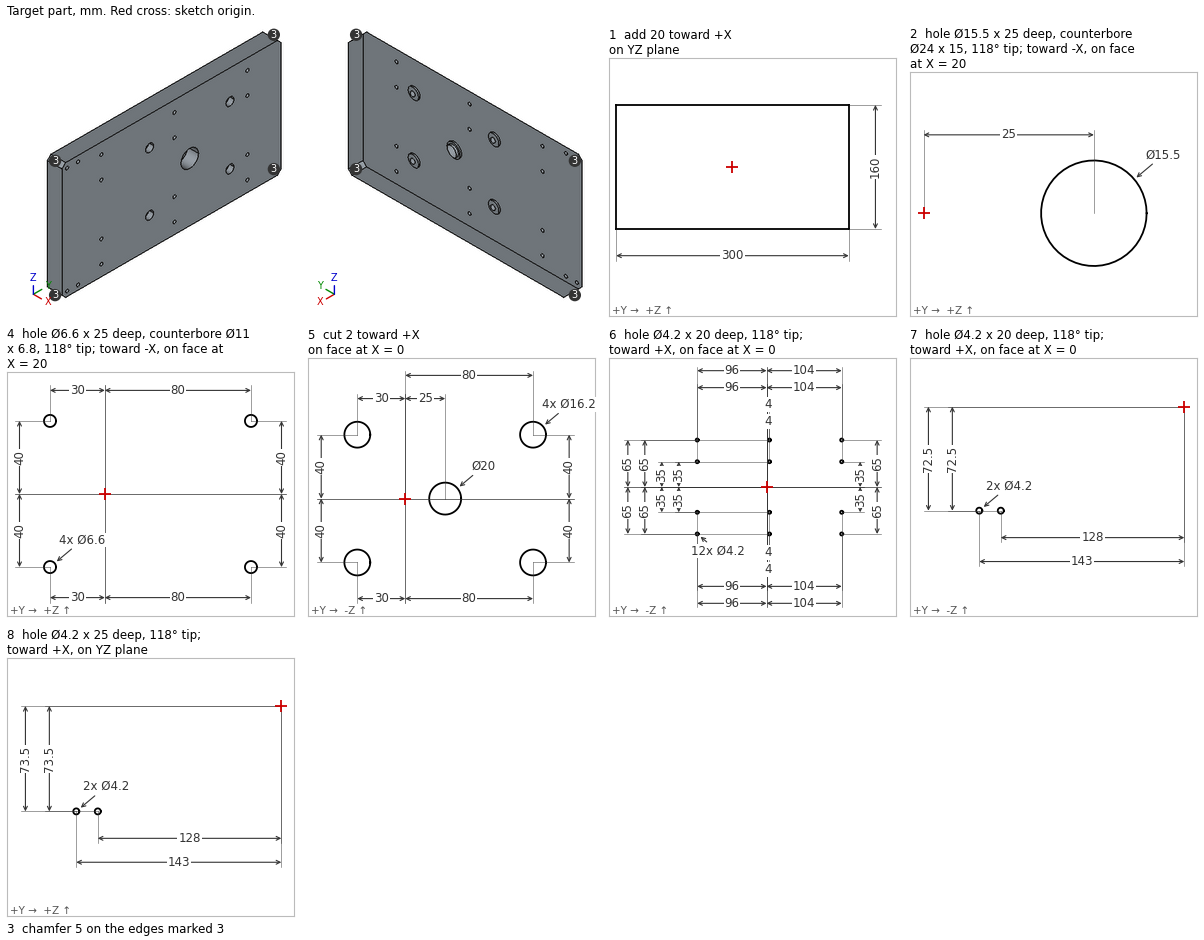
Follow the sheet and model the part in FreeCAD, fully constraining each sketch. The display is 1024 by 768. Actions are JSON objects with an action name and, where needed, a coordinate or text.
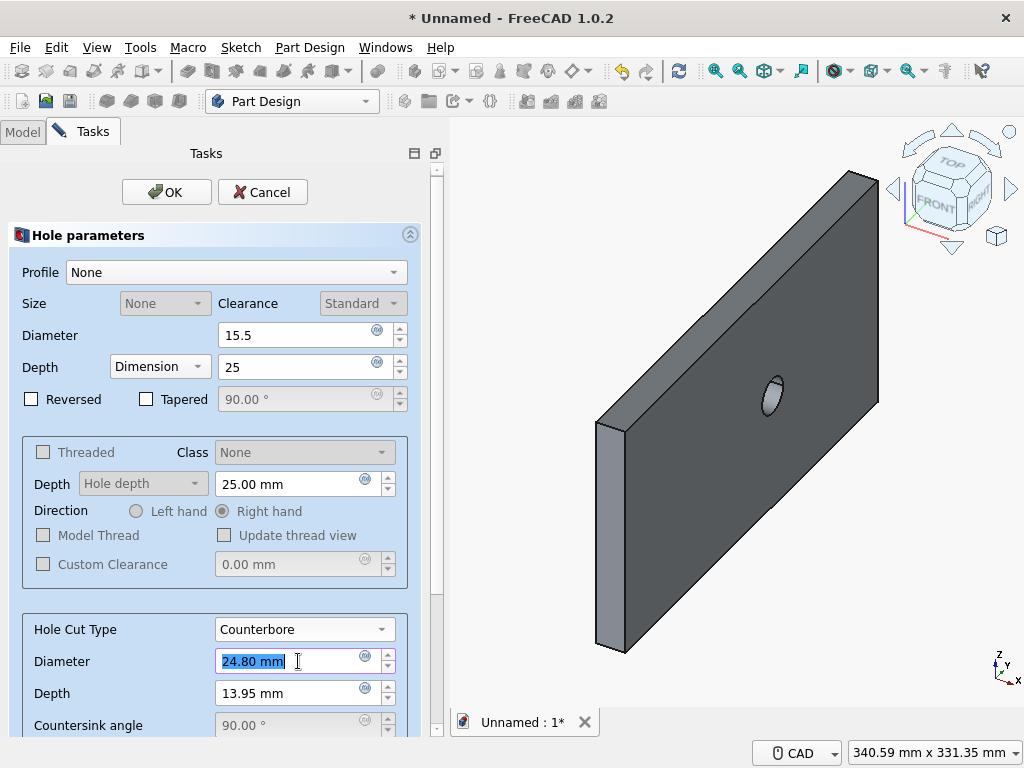
{"action": "type", "text": "24"}
{"action": "key", "text": "Tab"}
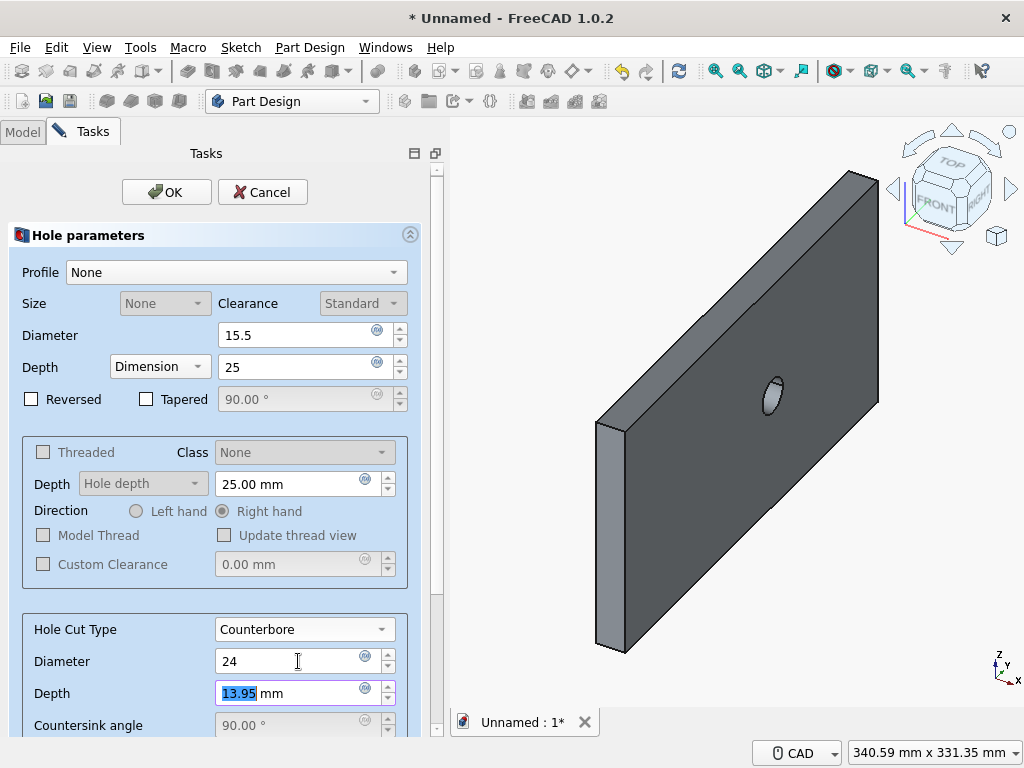
{"action": "type", "text": "15"}
{"action": "key", "text": "Tab"}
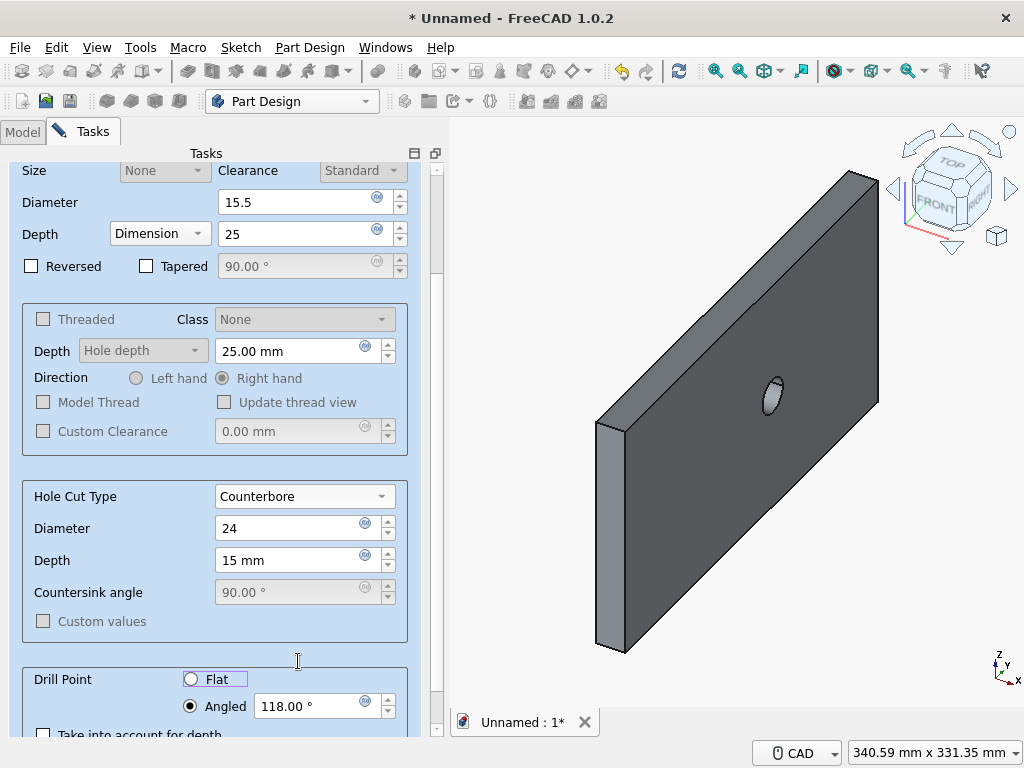
{"action": "scroll", "coordinate": [437, 450], "scroll_direction": "up", "scroll_amount": 3}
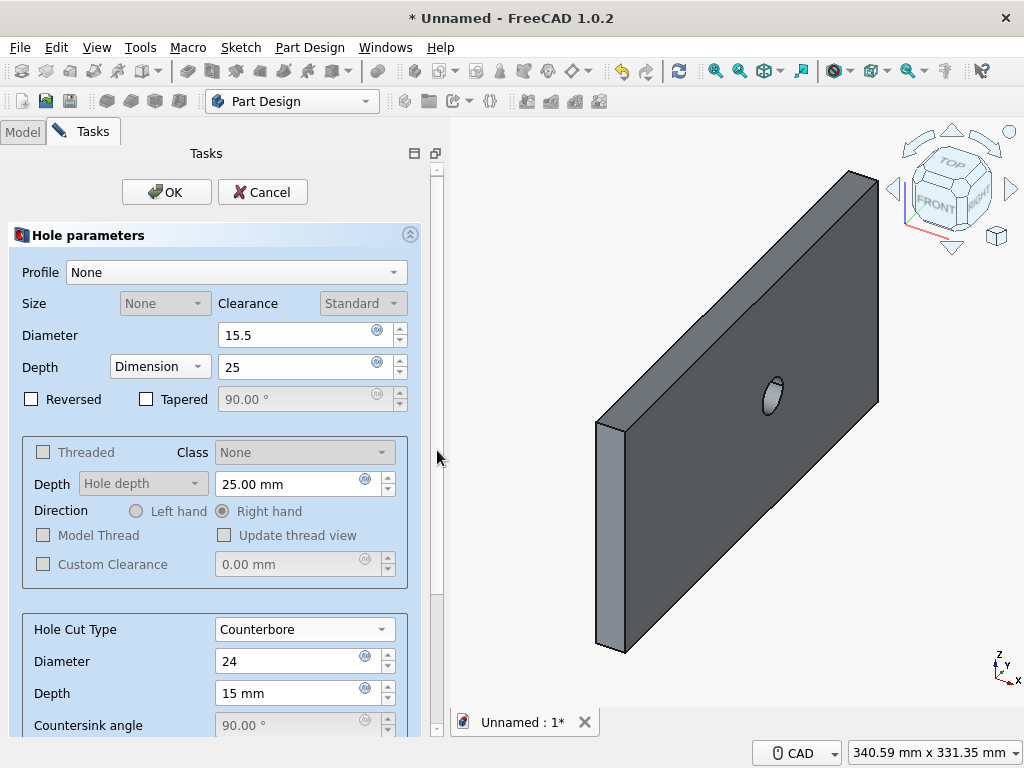
{"action": "left_click", "coordinate": [167, 192]}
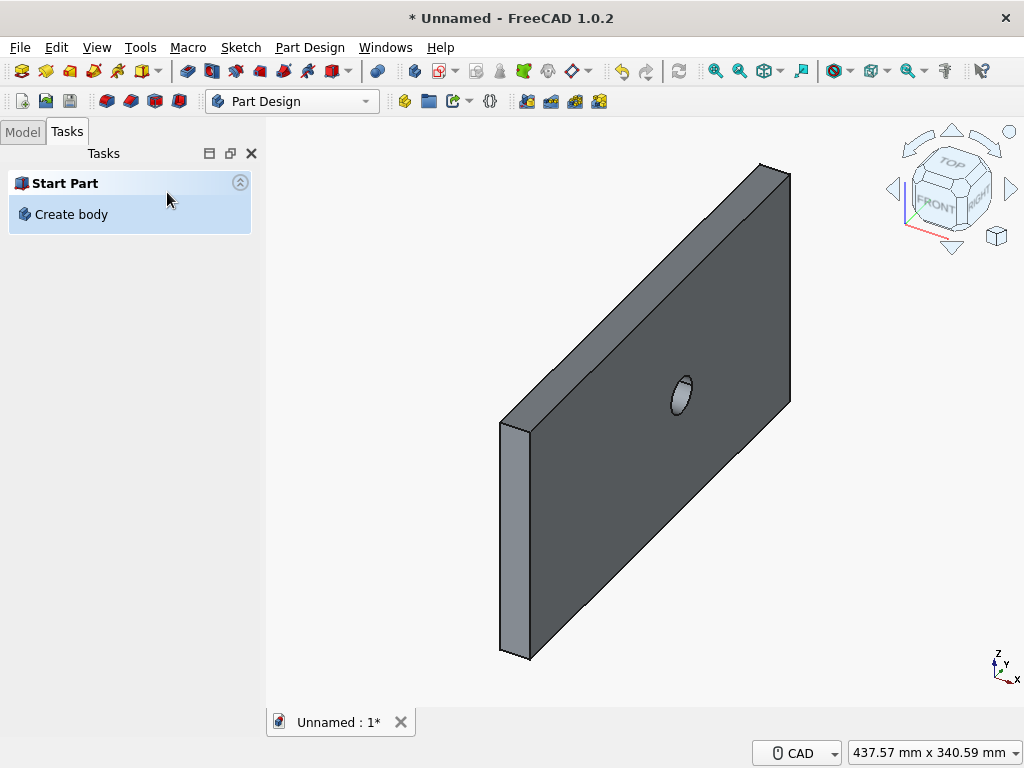
{"action": "left_click", "coordinate": [515, 427]}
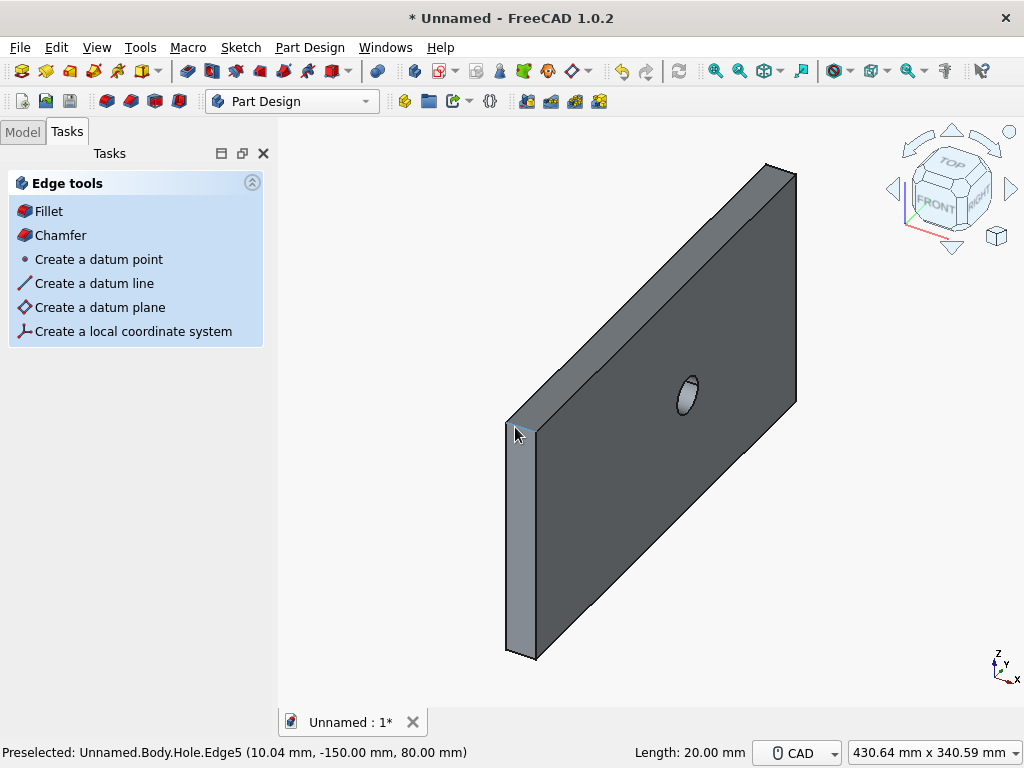
{"action": "key", "text": "0"}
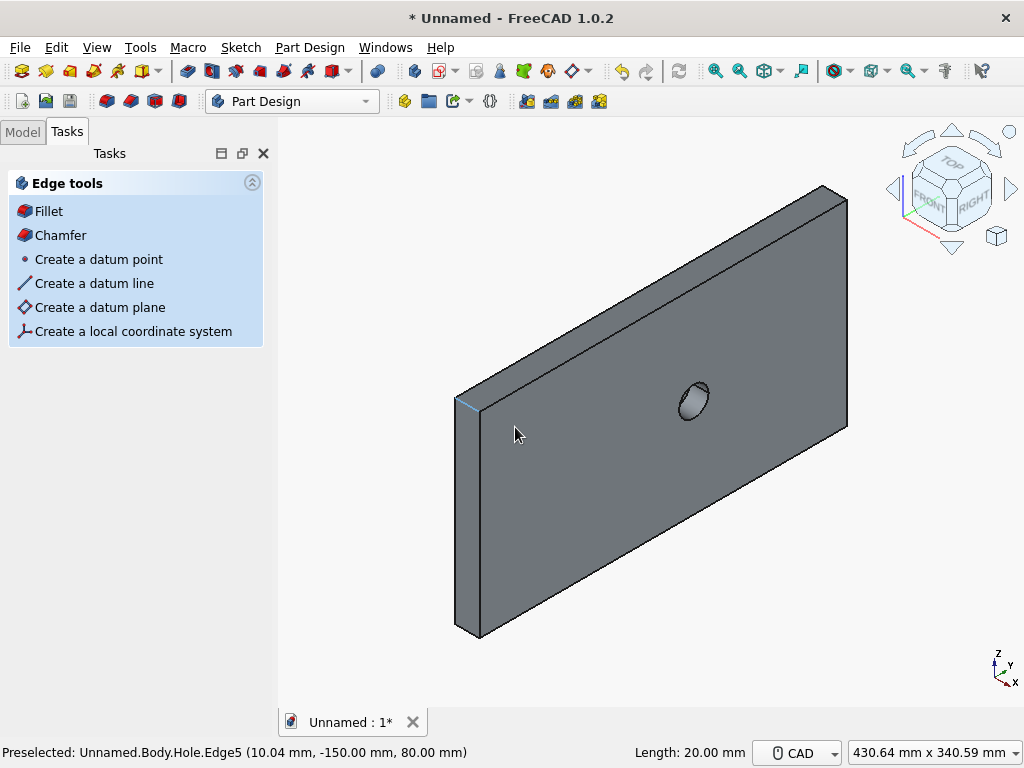
{"action": "key", "text": "2"}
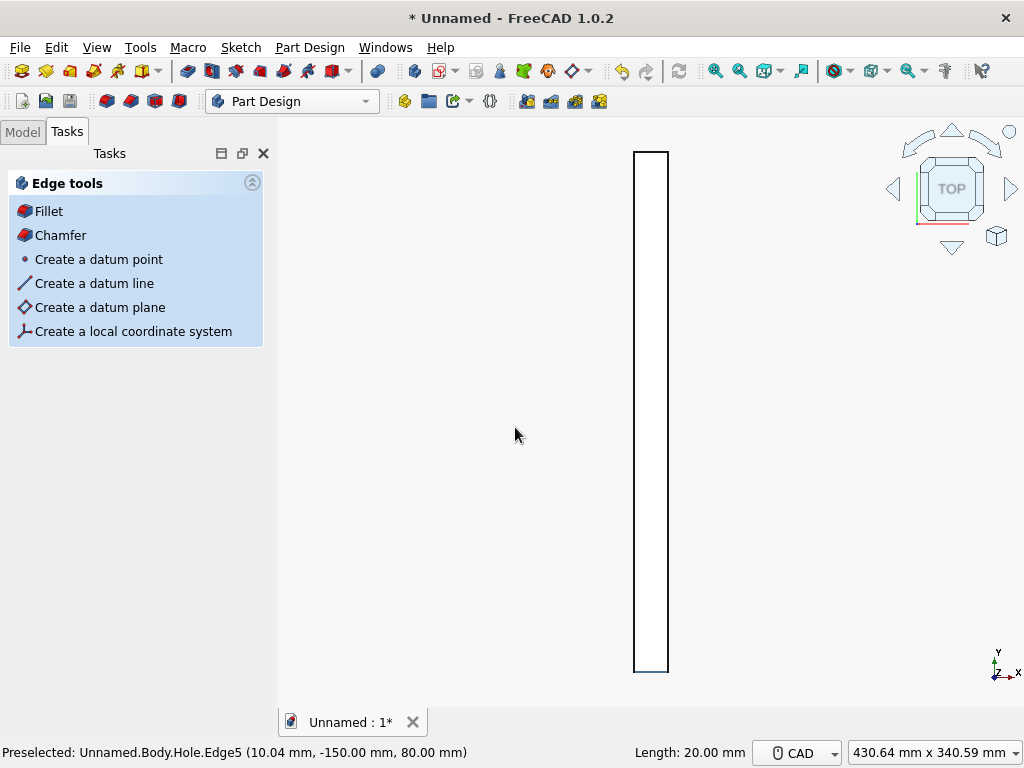
{"action": "left_click", "coordinate": [651, 151], "text": "ctrl"}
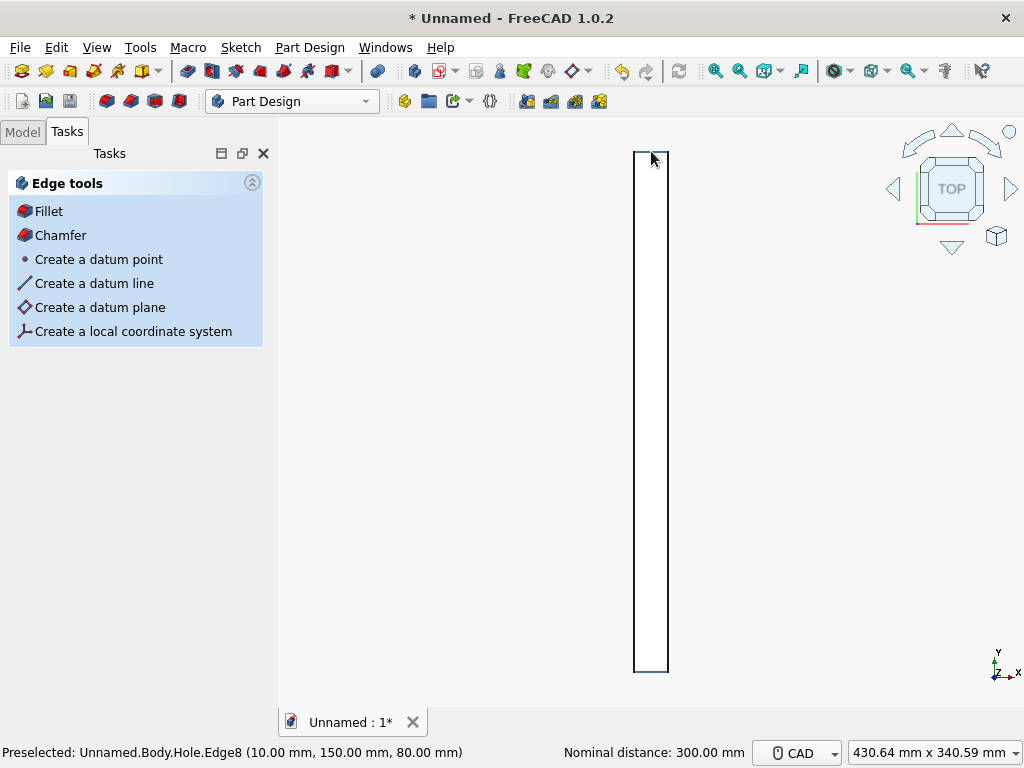
{"action": "key", "text": "1"}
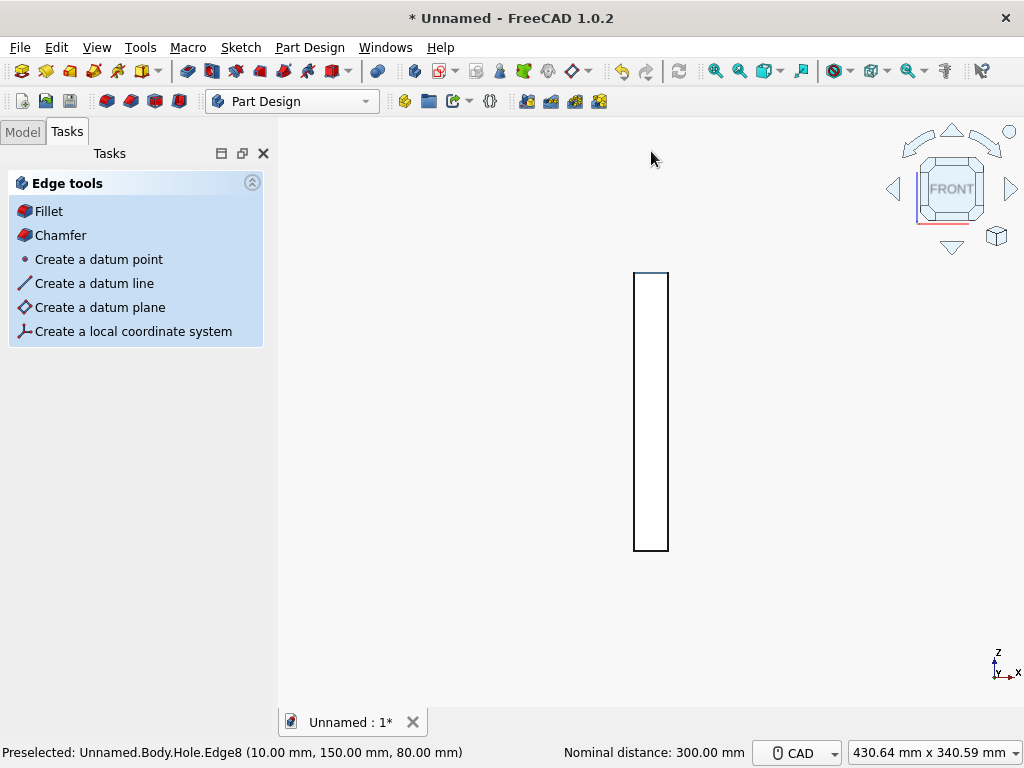
{"action": "left_click", "coordinate": [651, 550], "text": "ctrl"}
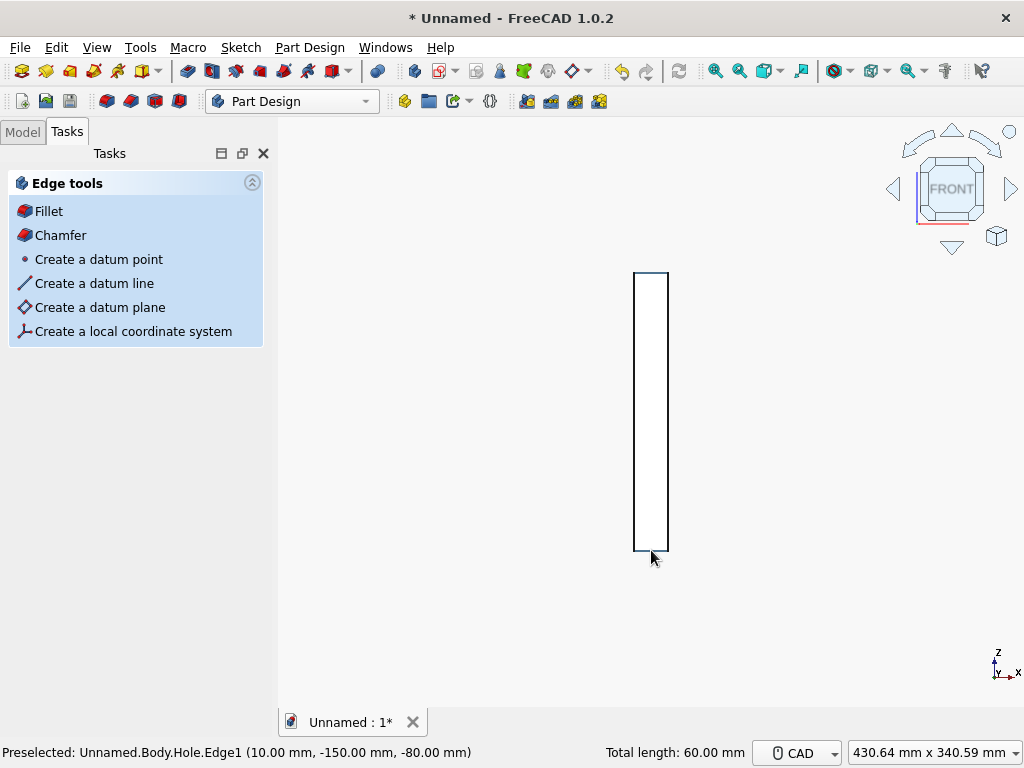
{"action": "key", "text": "3"}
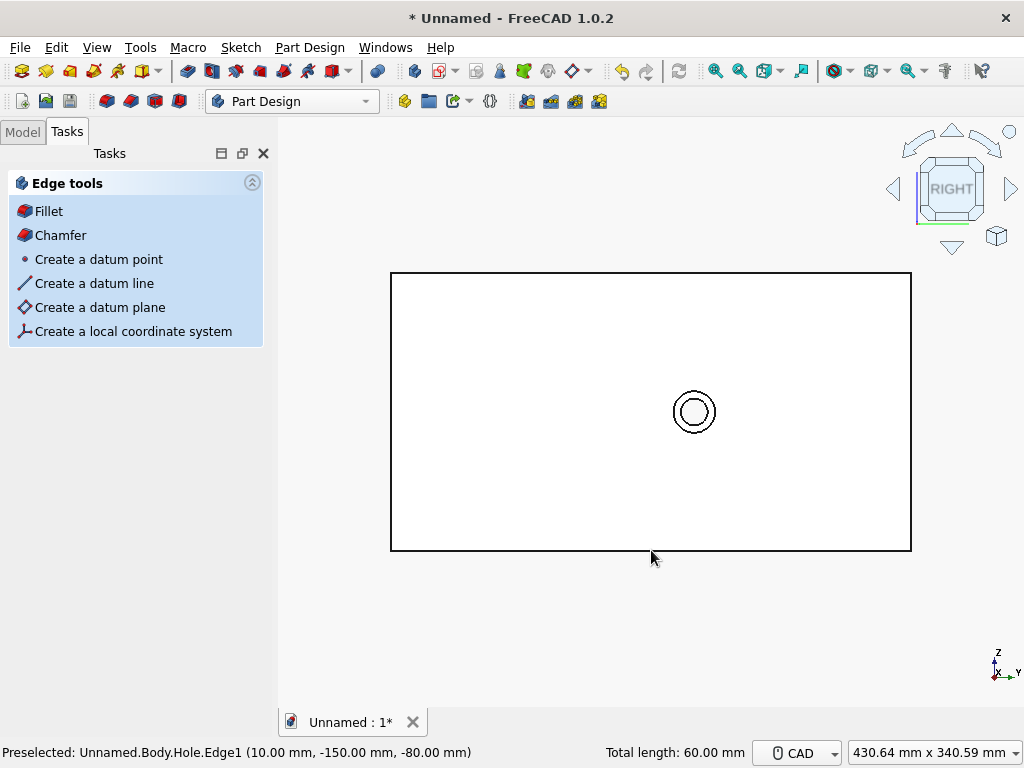
{"action": "key", "text": "5"}